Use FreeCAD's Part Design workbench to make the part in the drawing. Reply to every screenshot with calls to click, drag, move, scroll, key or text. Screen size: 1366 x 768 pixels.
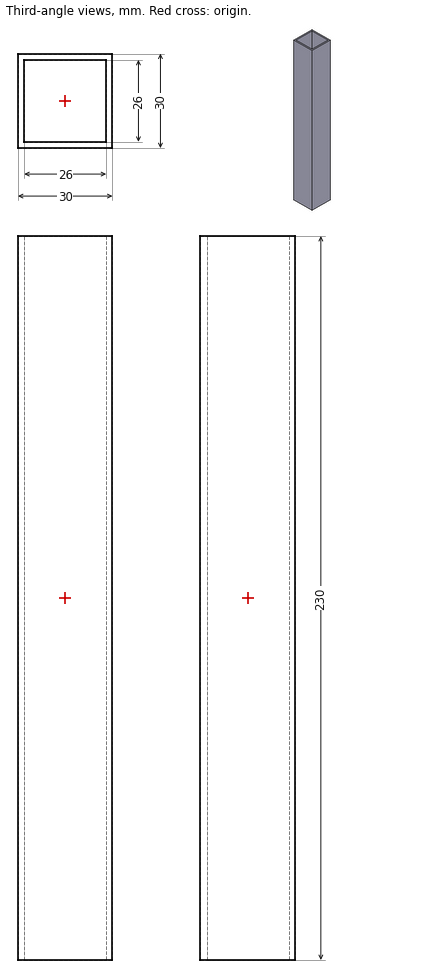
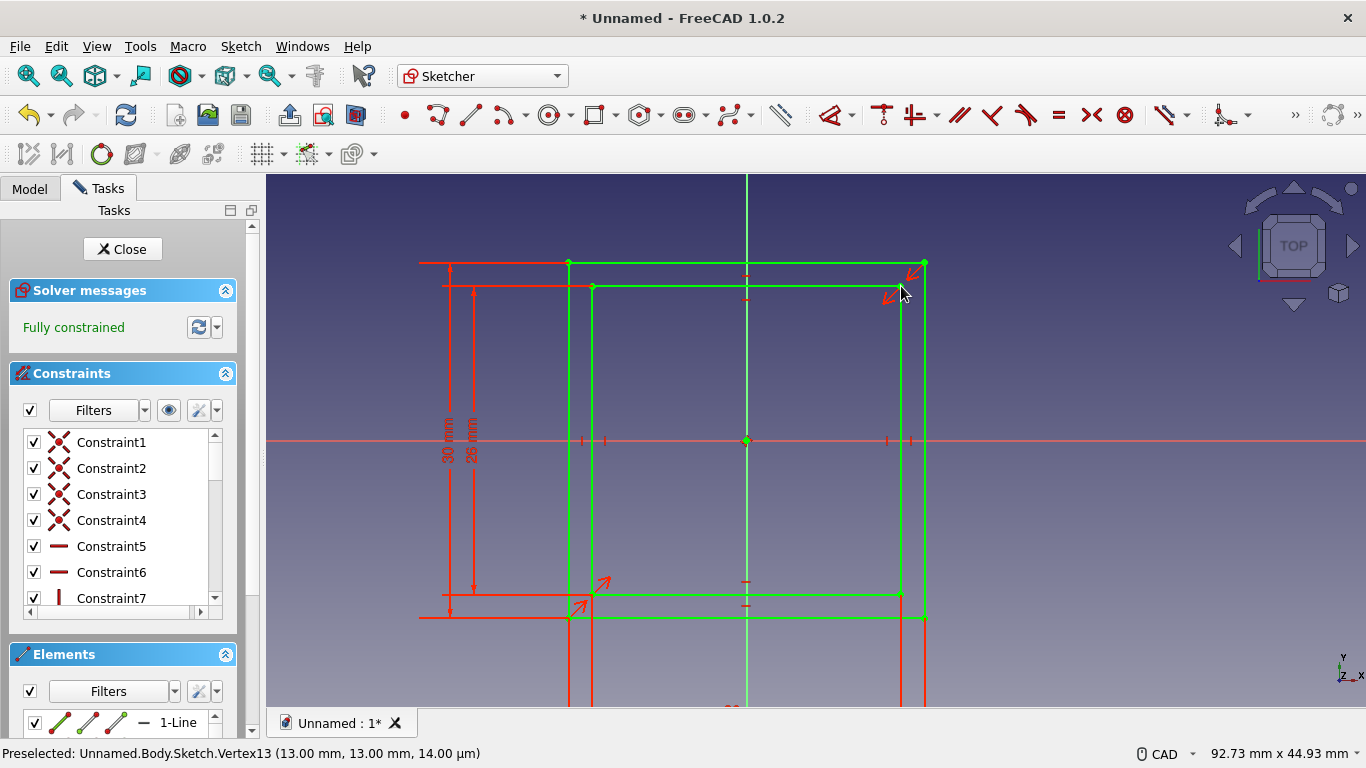
click(123, 249)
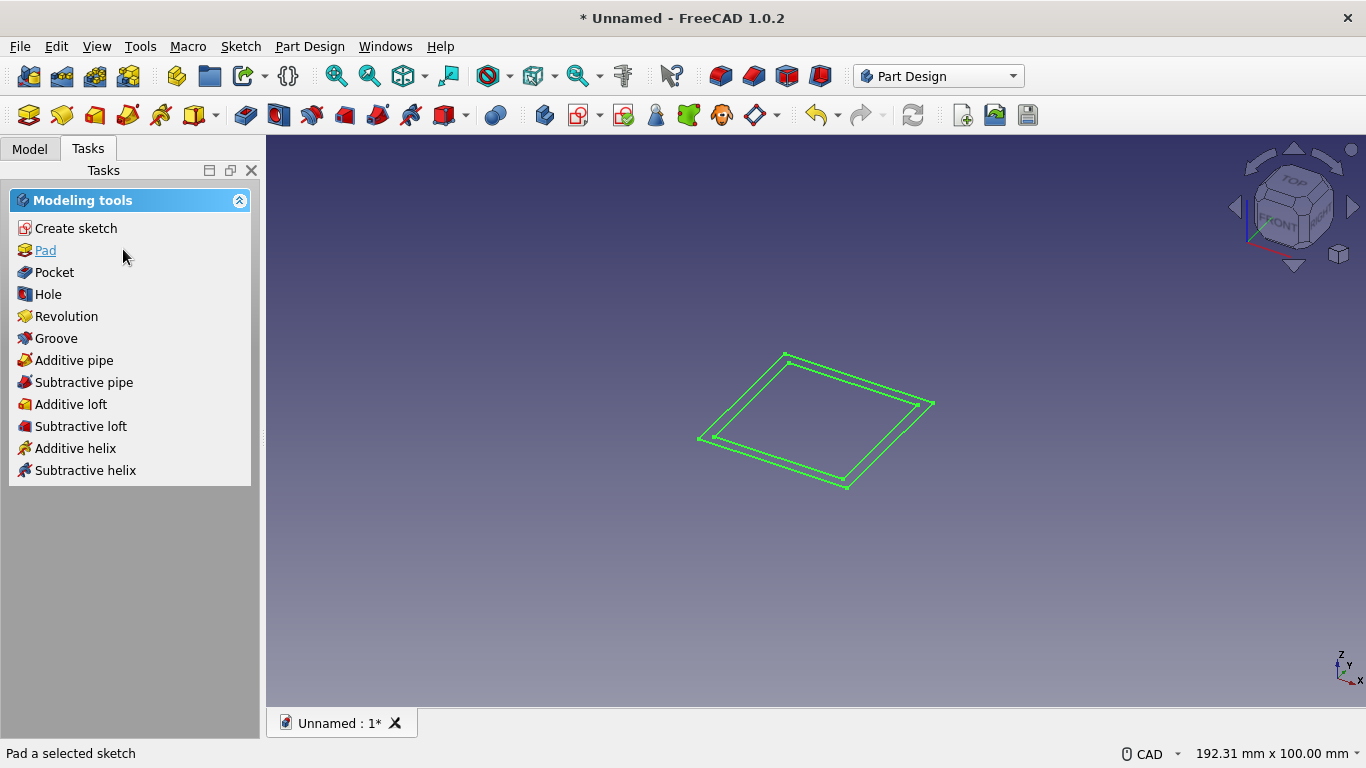
click(29, 116)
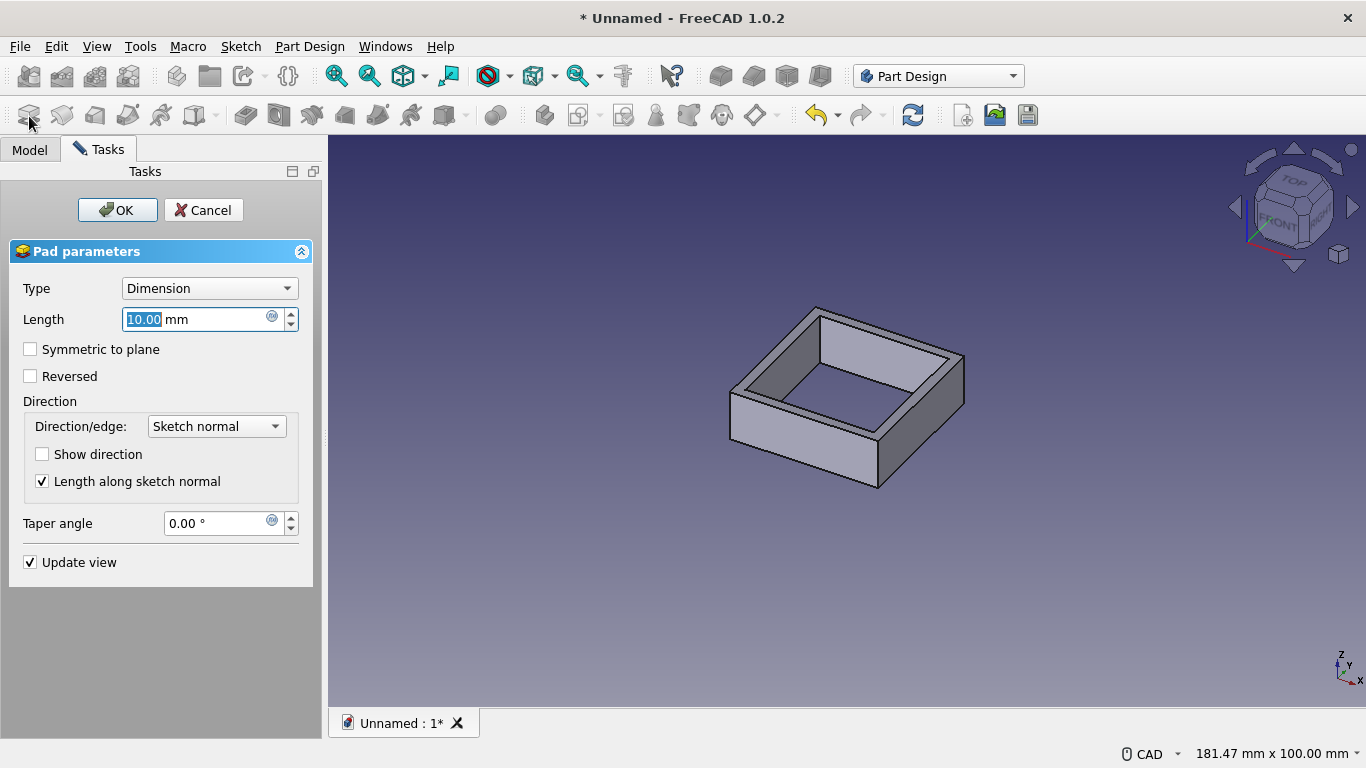
text(230)
key(Tab)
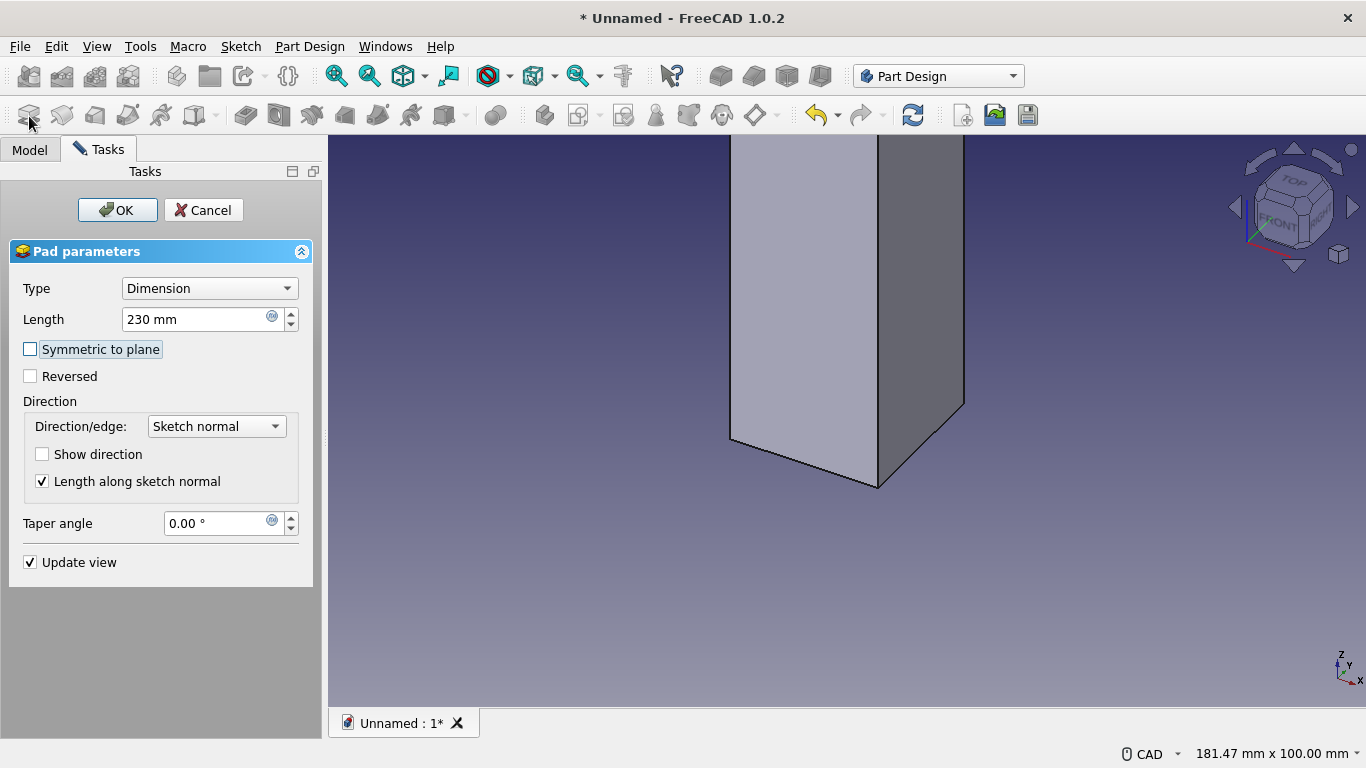
click(31, 349)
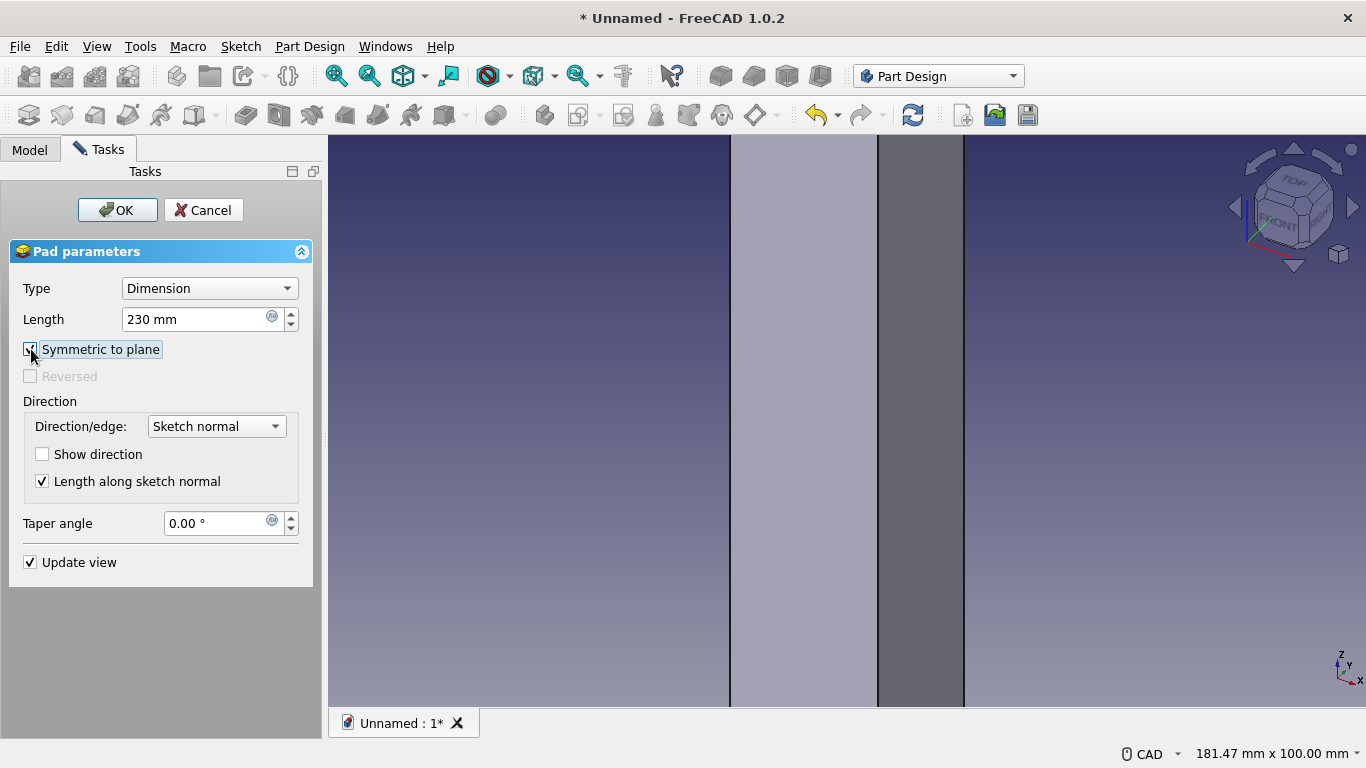
click(118, 210)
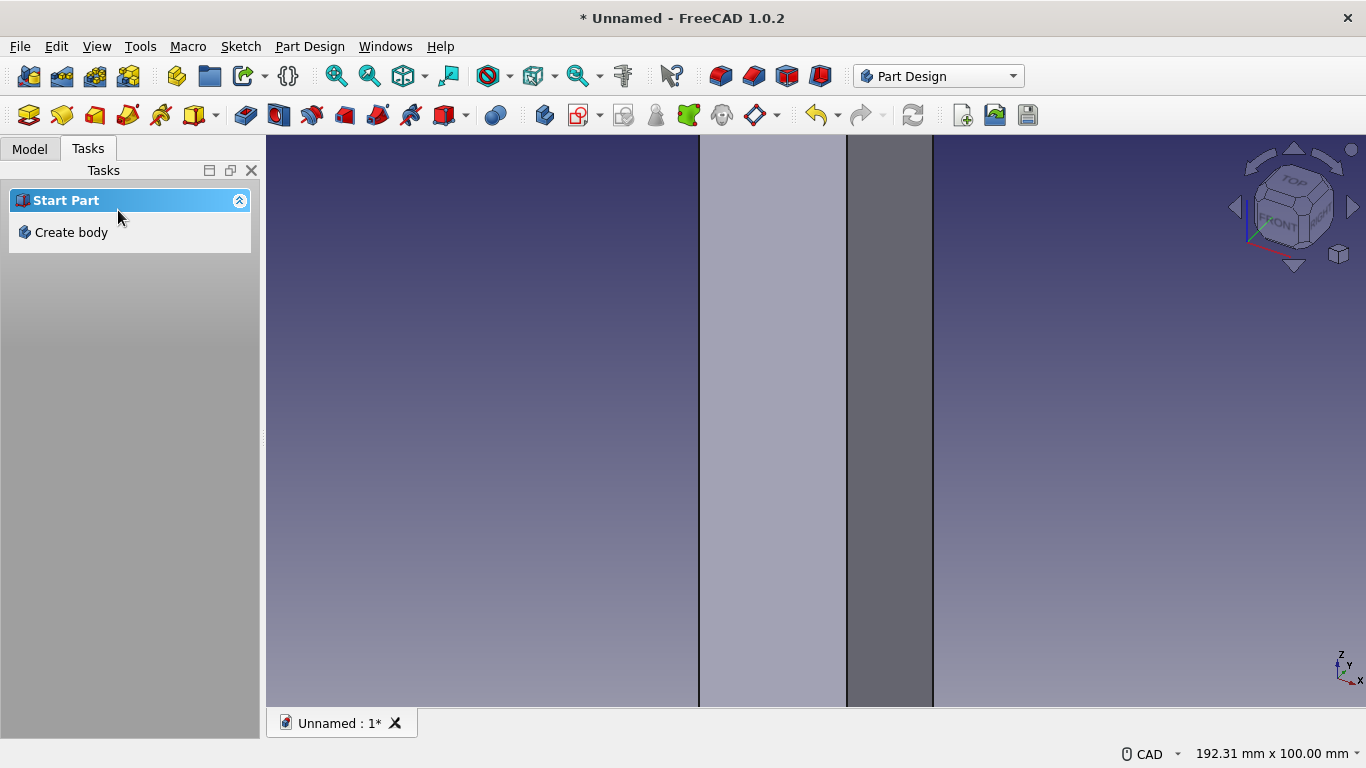
key(0)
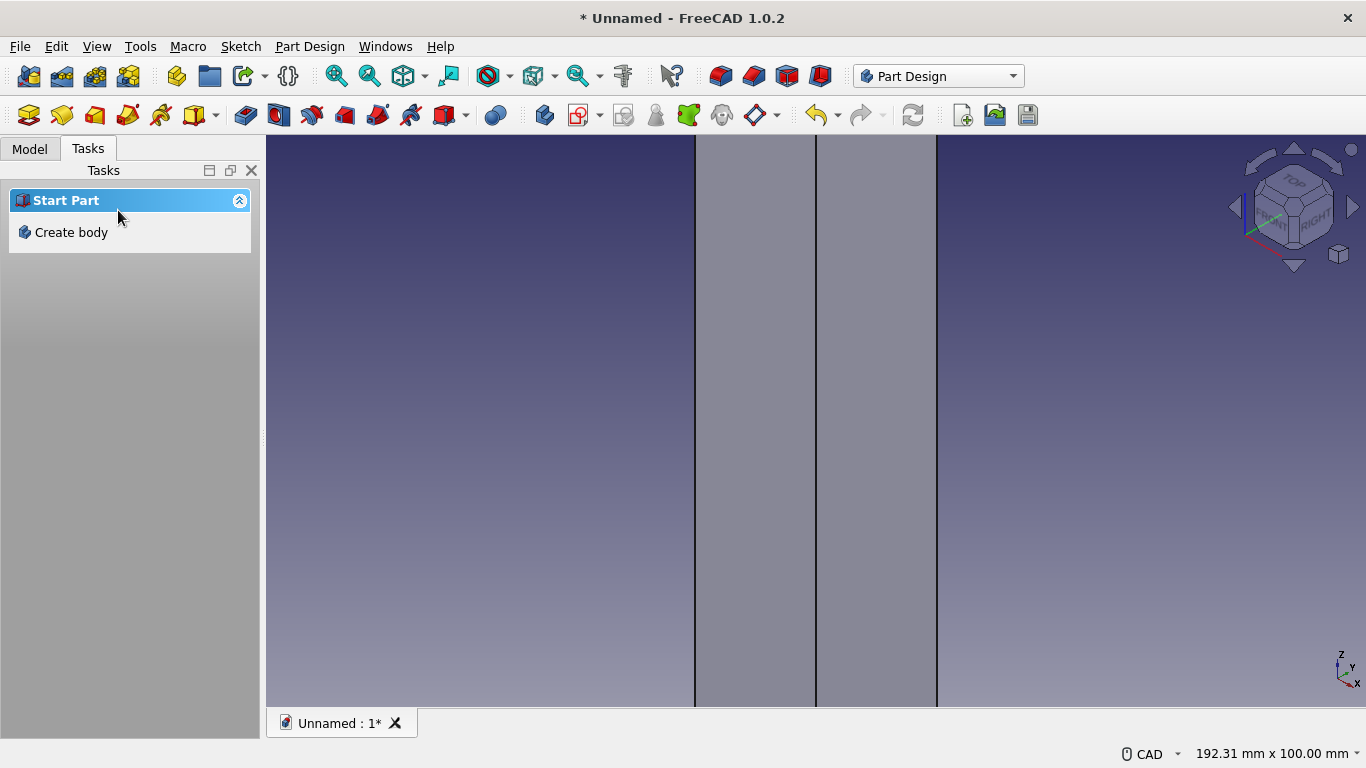
click(337, 76)